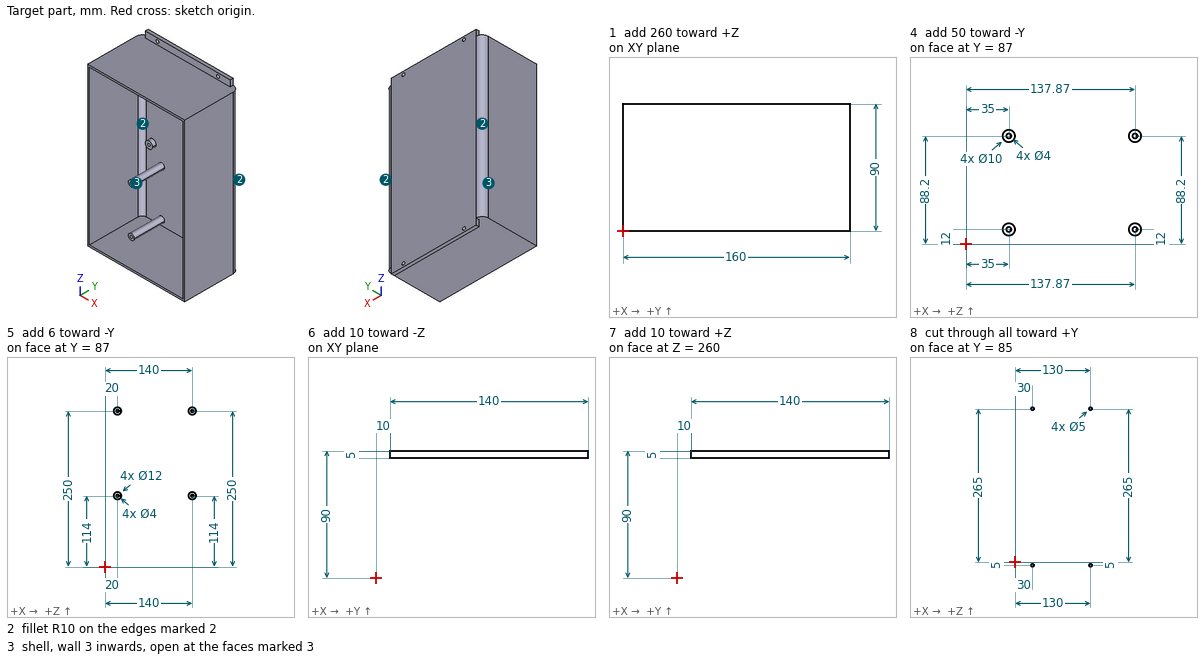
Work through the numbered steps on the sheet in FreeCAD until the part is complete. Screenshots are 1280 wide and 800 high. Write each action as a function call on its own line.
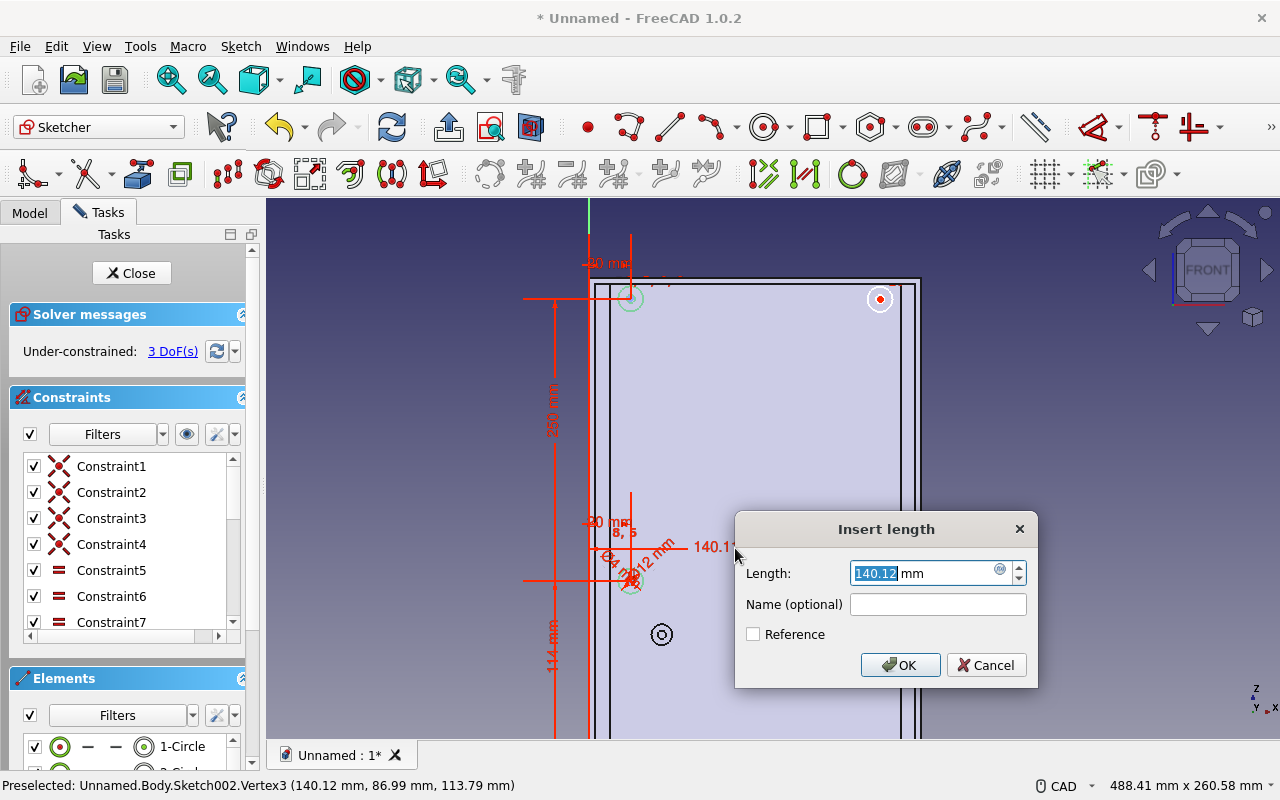
text(140)
key(Return)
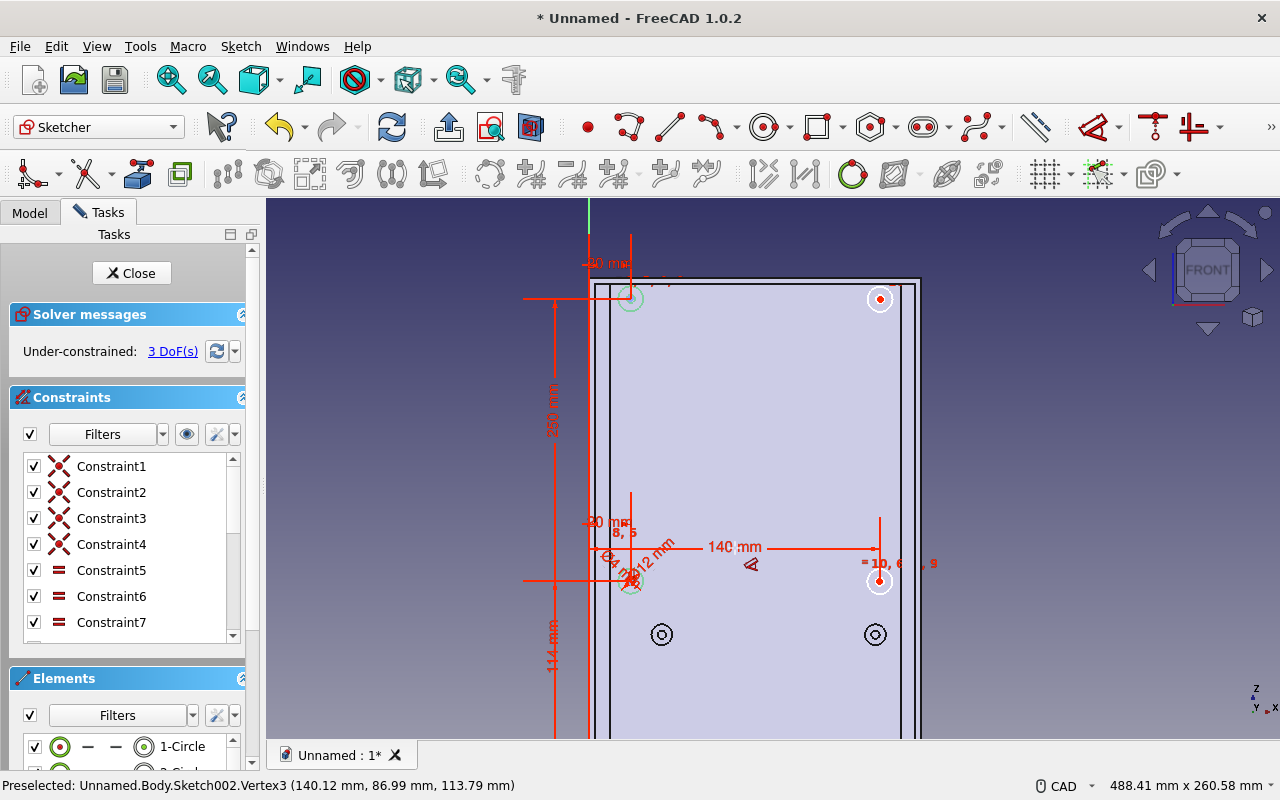
click(880, 582)
click(555, 617)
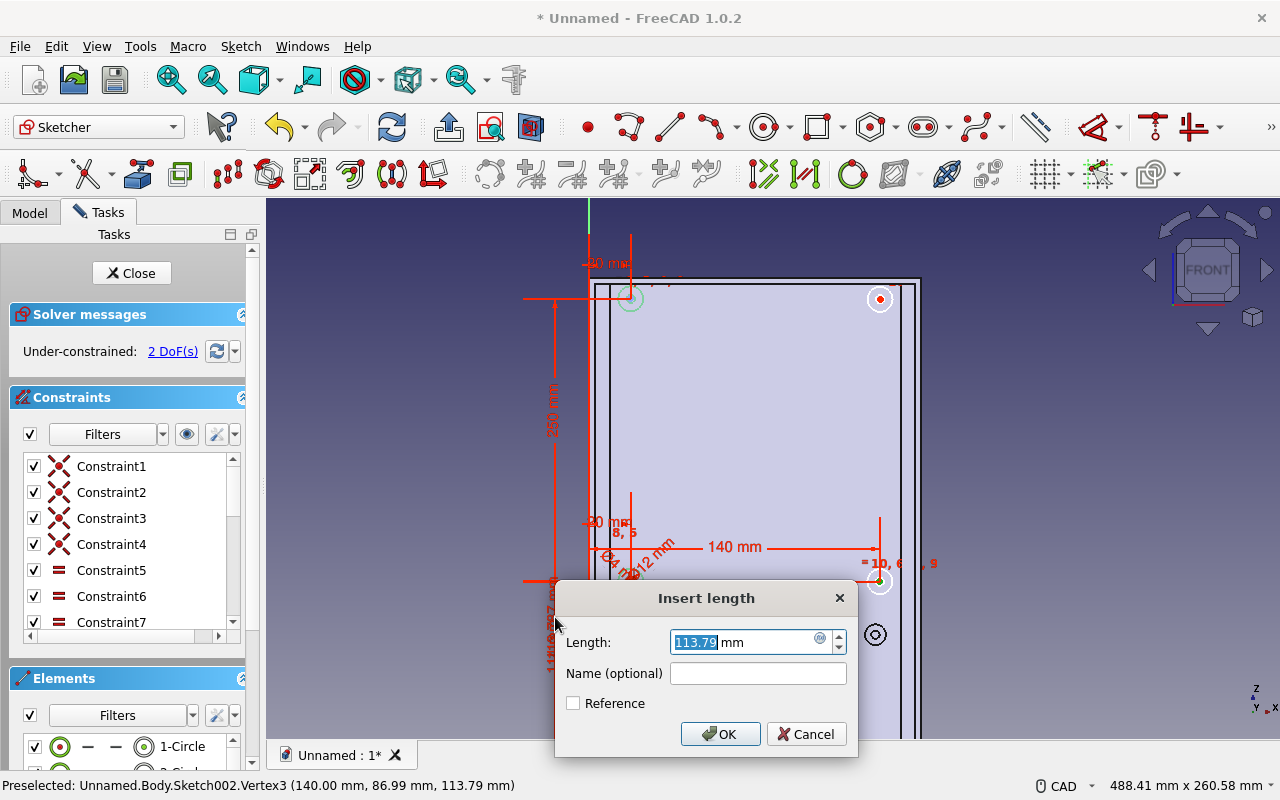
text(114)
key(Return)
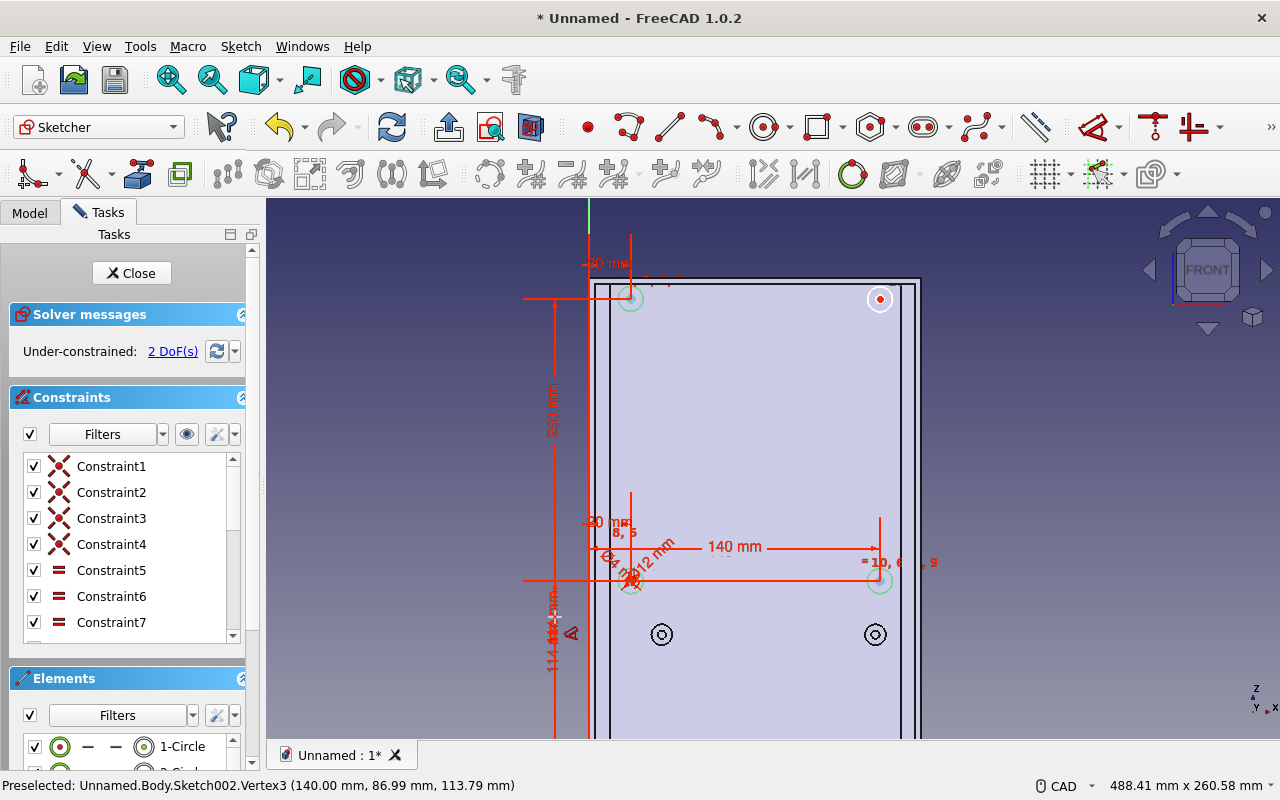
click(880, 299)
click(735, 265)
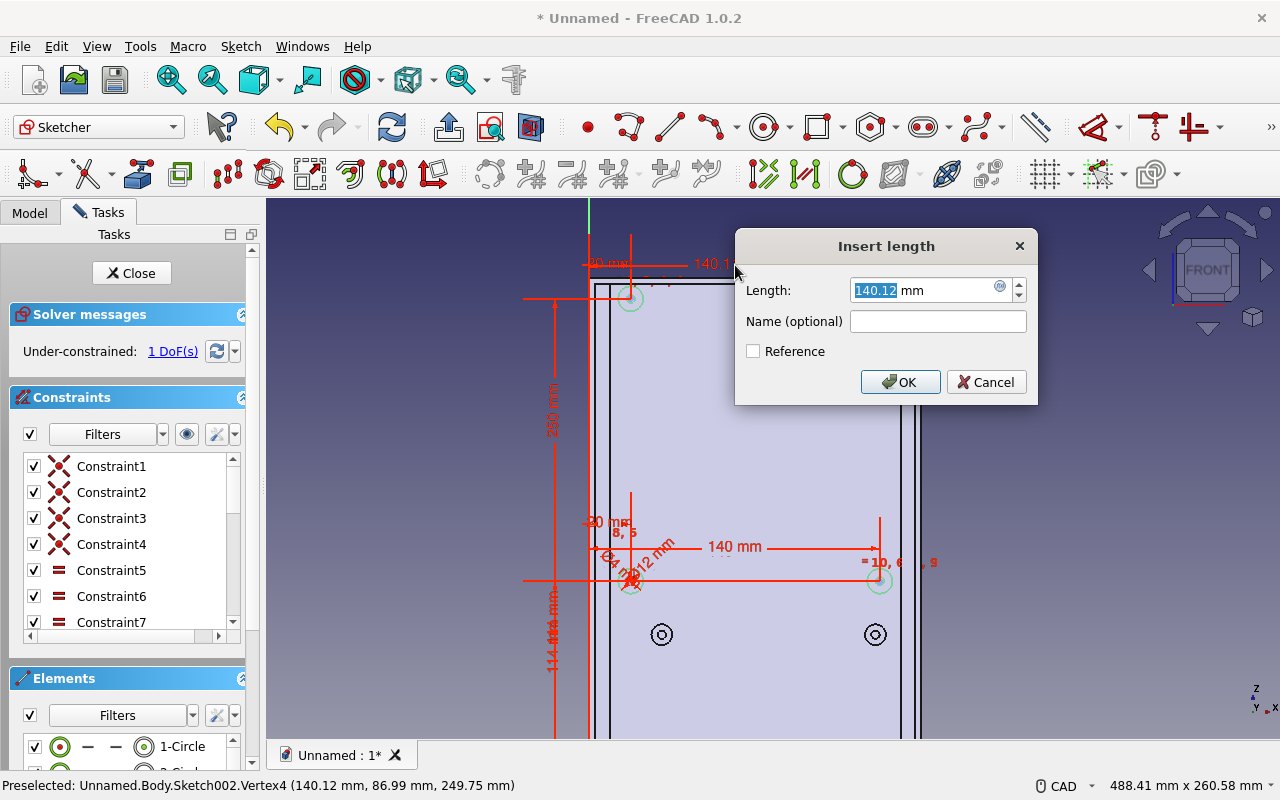
text(140)
key(Return)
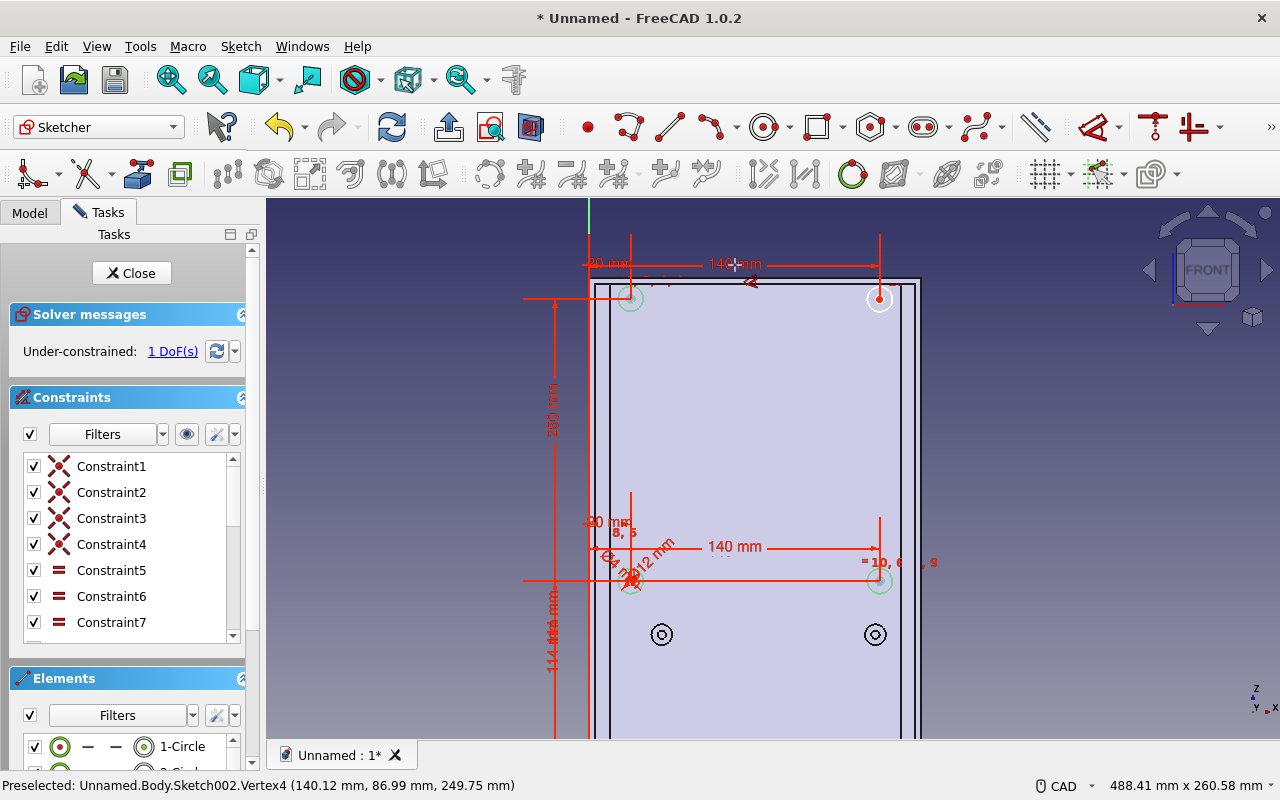
click(880, 299)
click(555, 361)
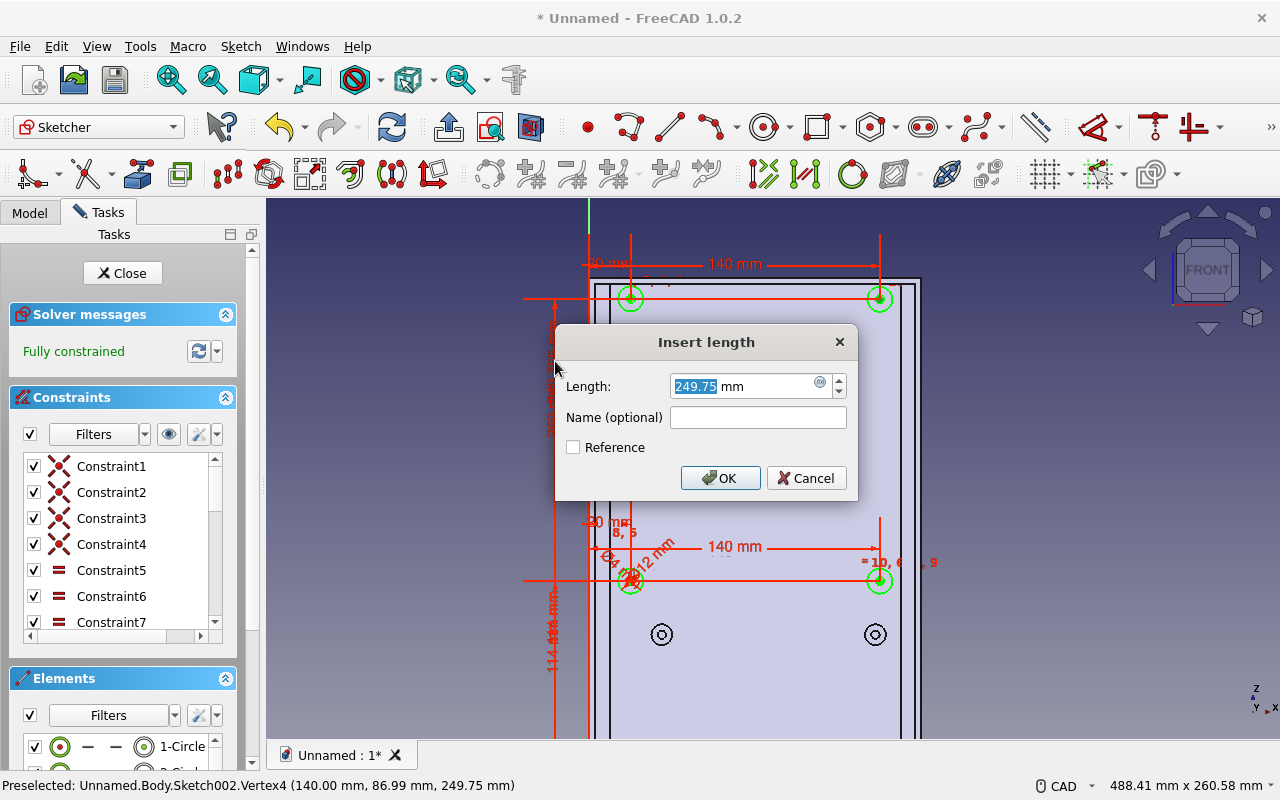
text(250)
key(Return)
key(Escape)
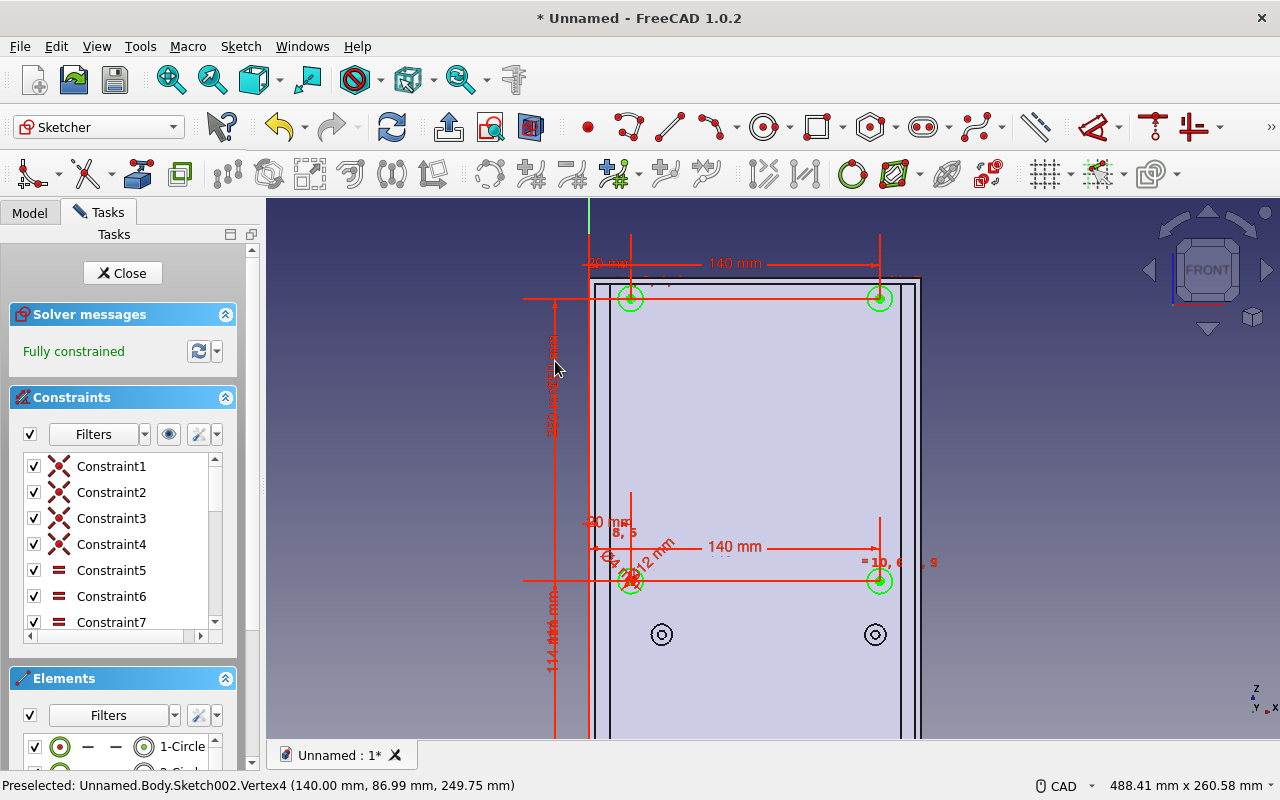
click(123, 273)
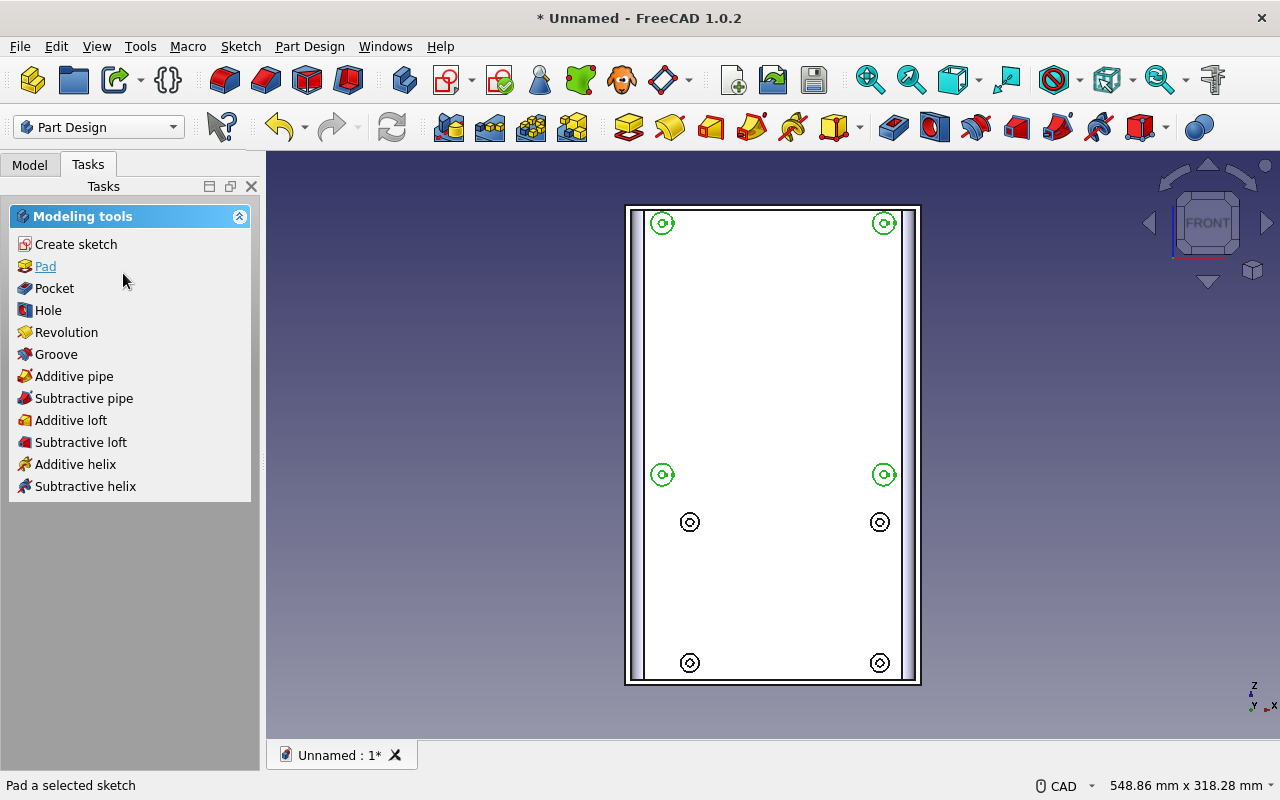
click(629, 128)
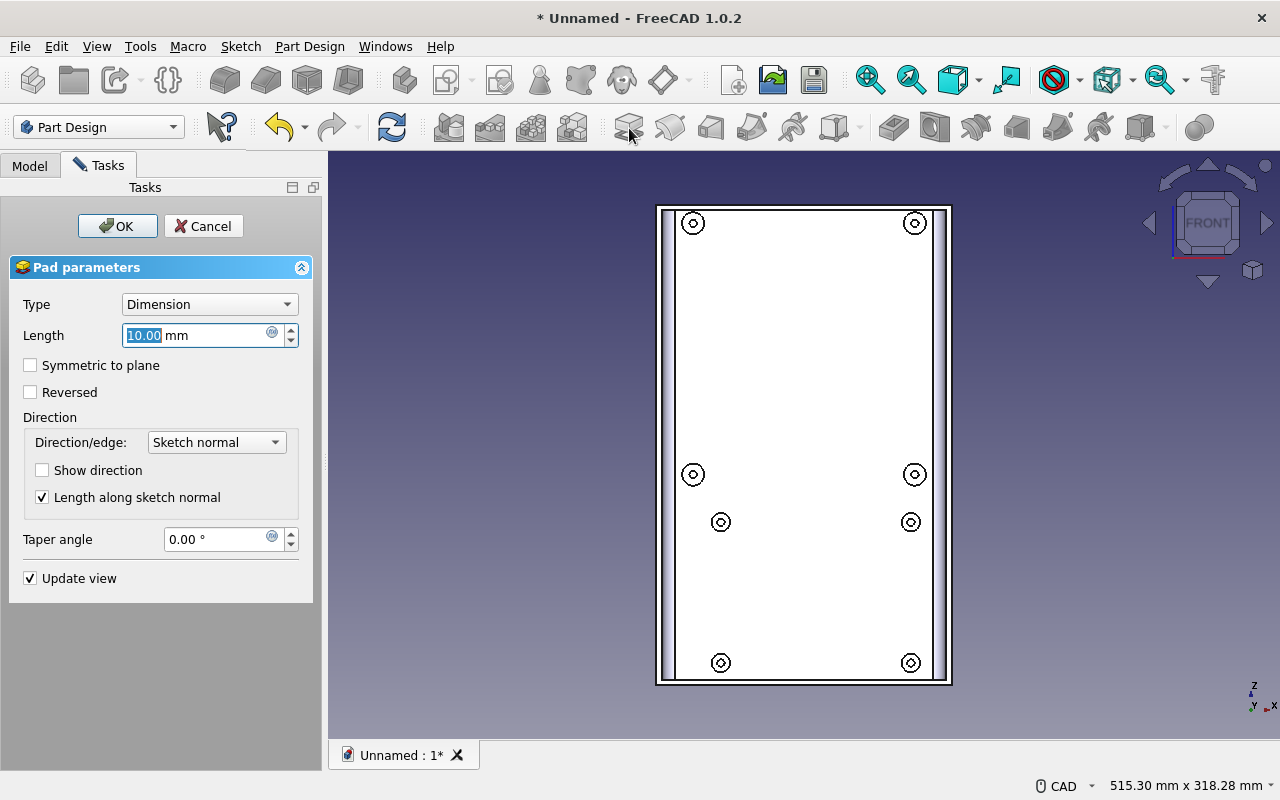
text(6)
key(Tab)